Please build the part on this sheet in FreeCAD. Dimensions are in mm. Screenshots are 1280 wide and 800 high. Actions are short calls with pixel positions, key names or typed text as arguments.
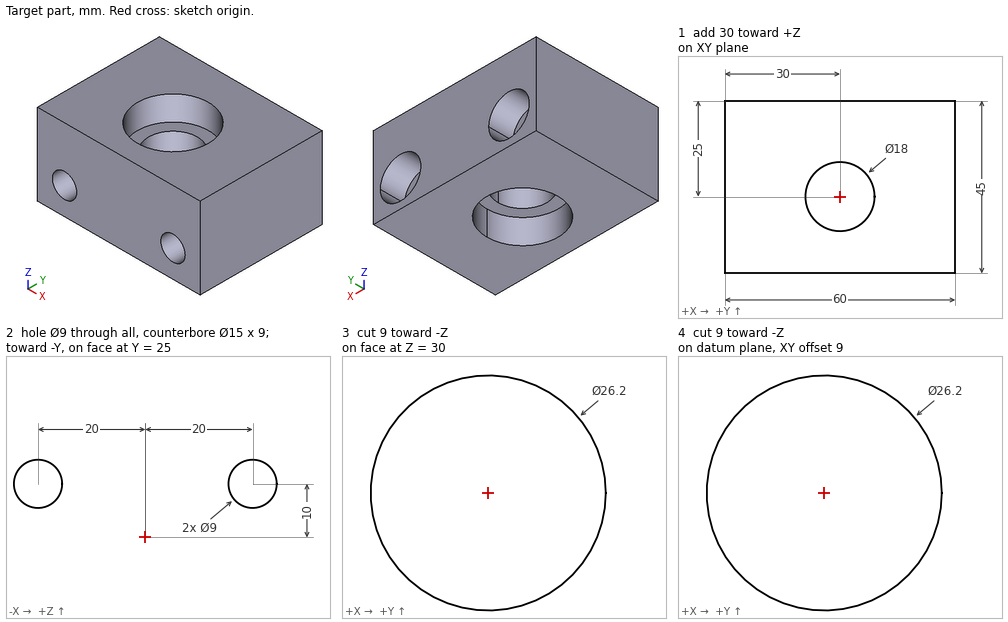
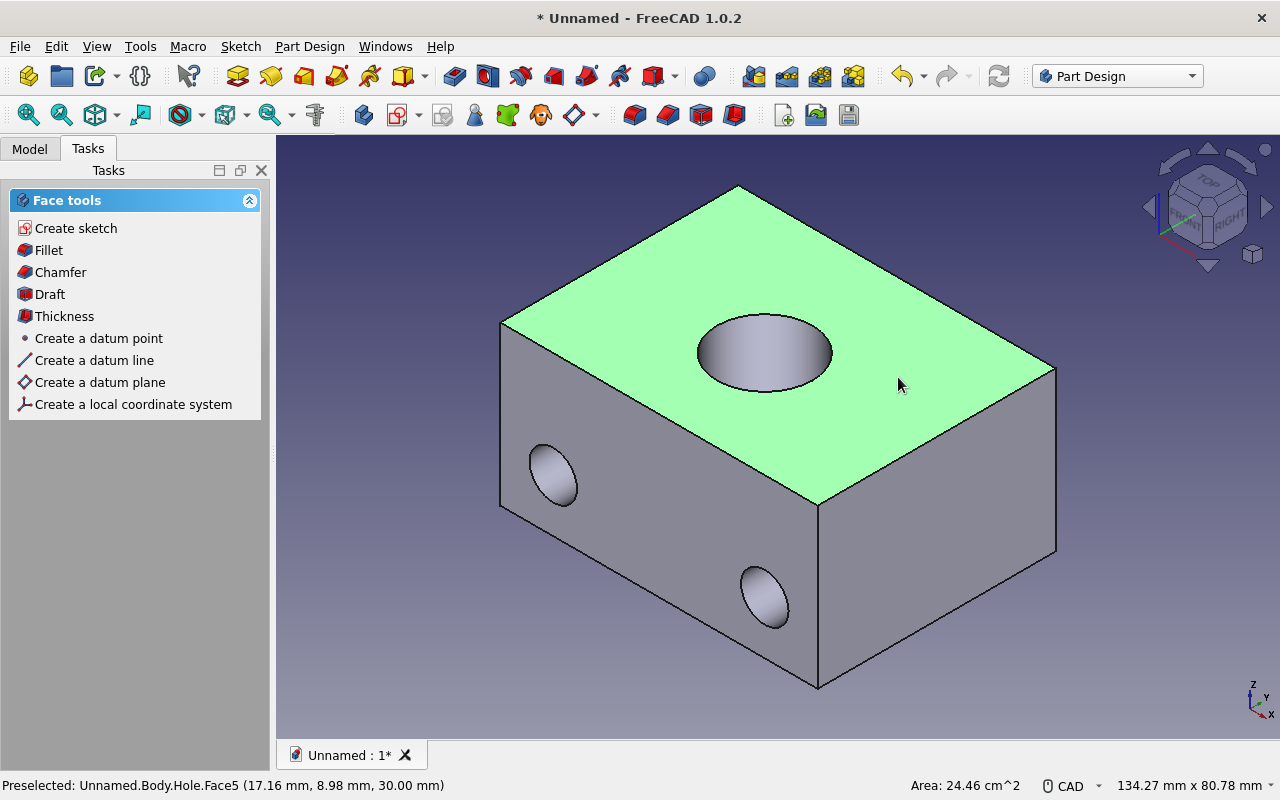
click(396, 116)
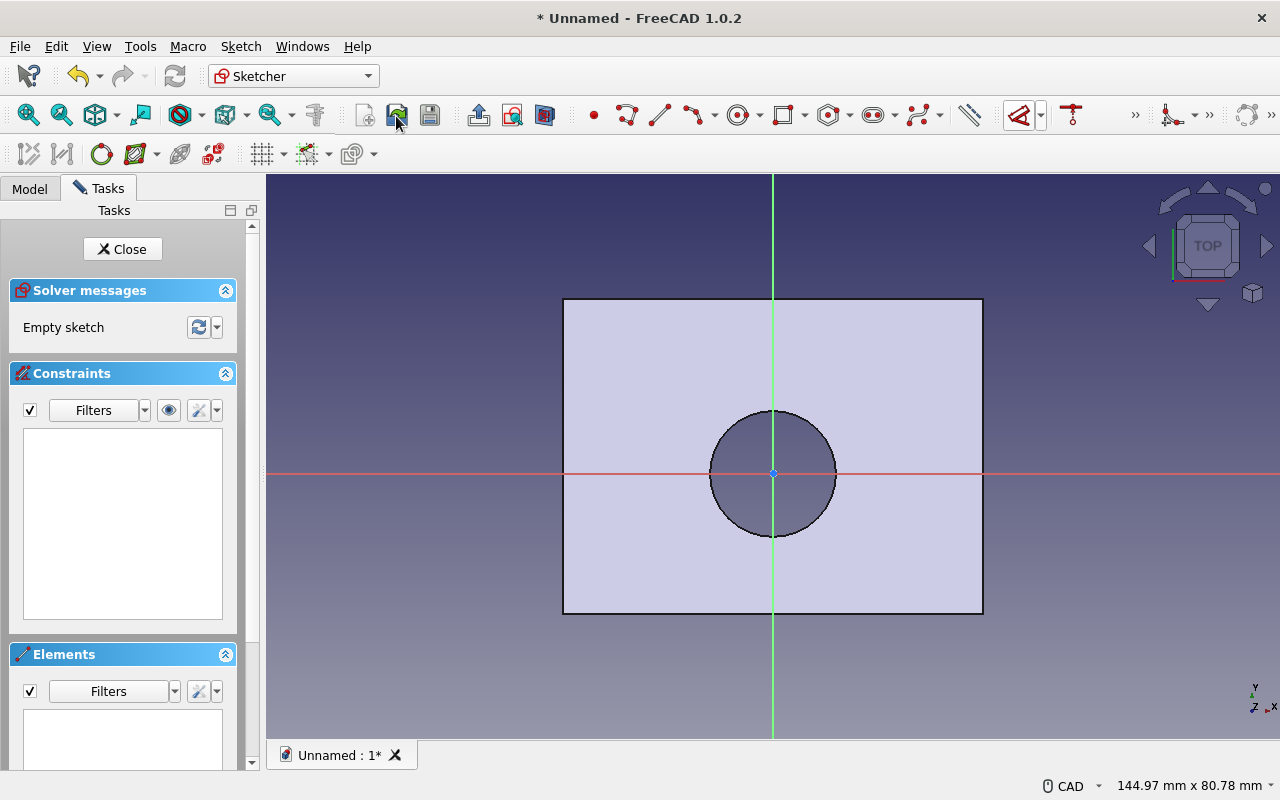
scroll(856, 495, up, 3)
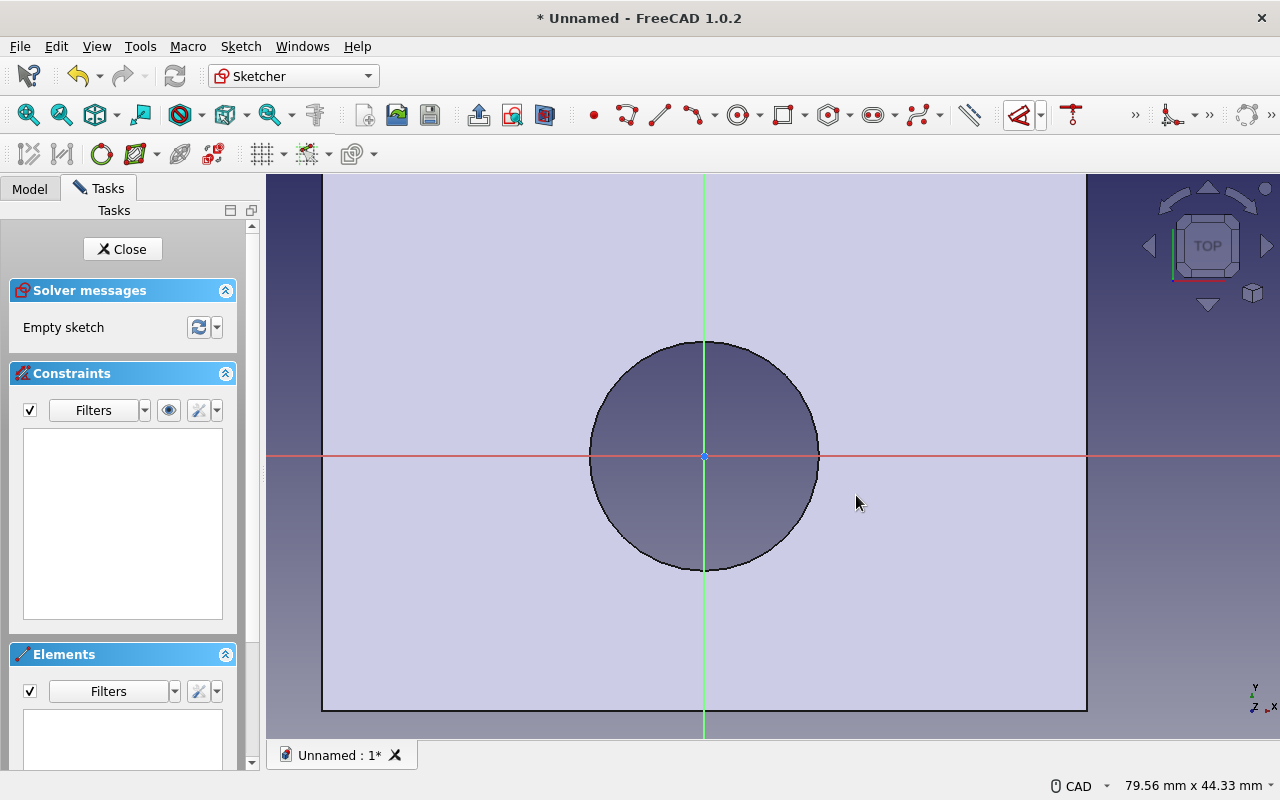
click(738, 116)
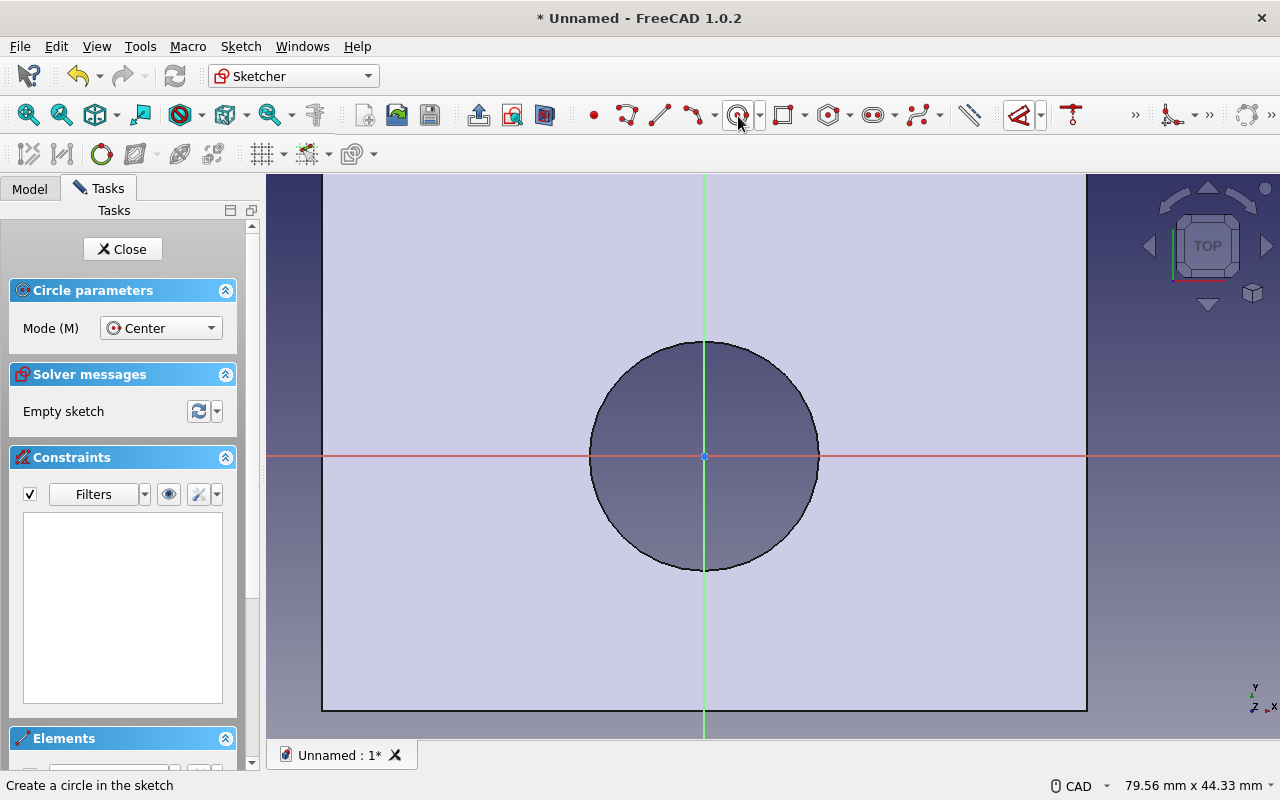
click(704, 456)
move(822, 338)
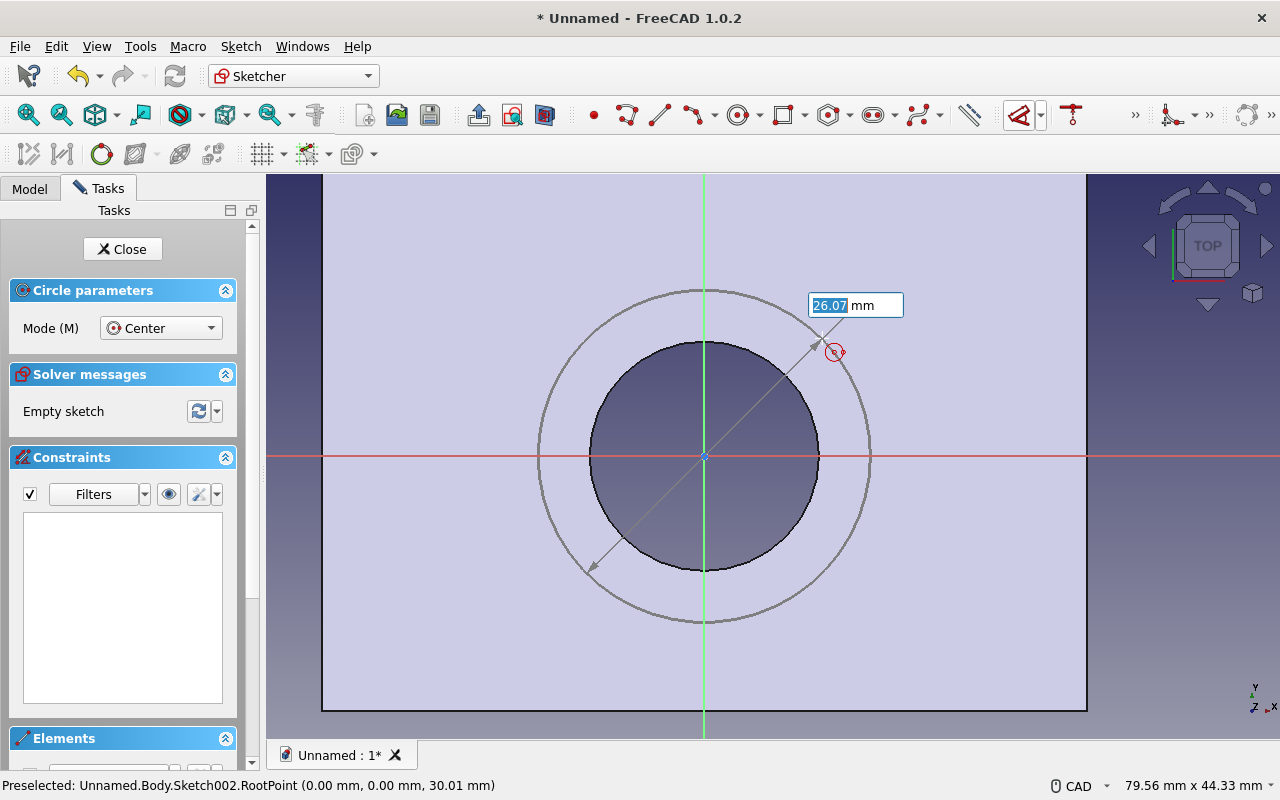
text(26.2)
key(Return)
key(Escape)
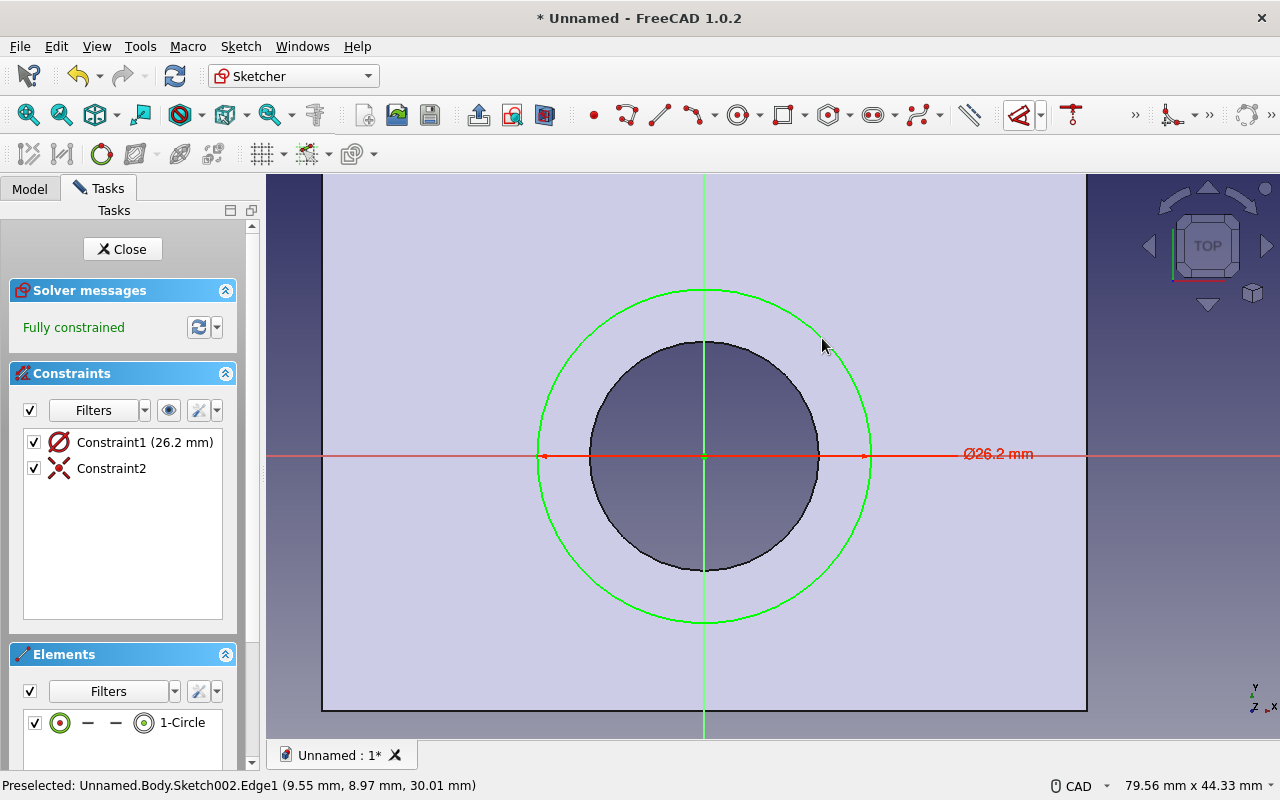
click(123, 249)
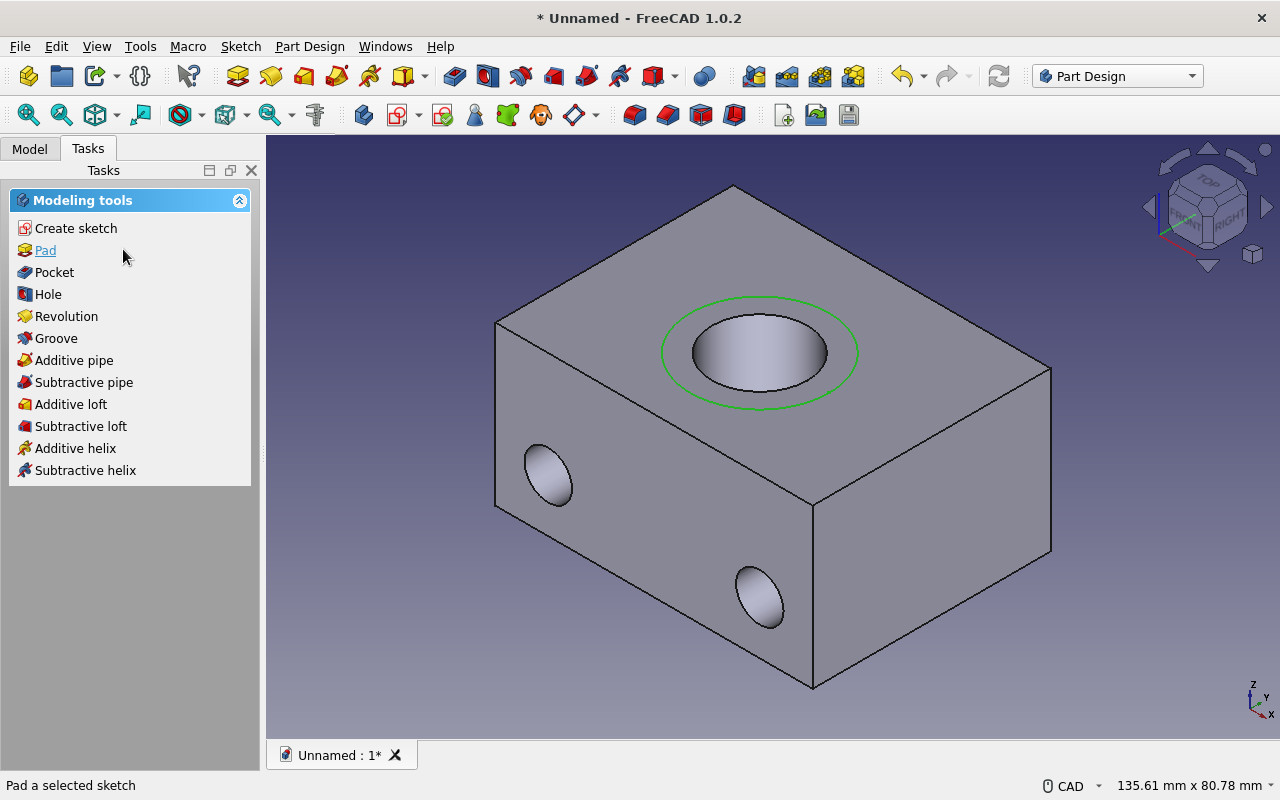
click(455, 76)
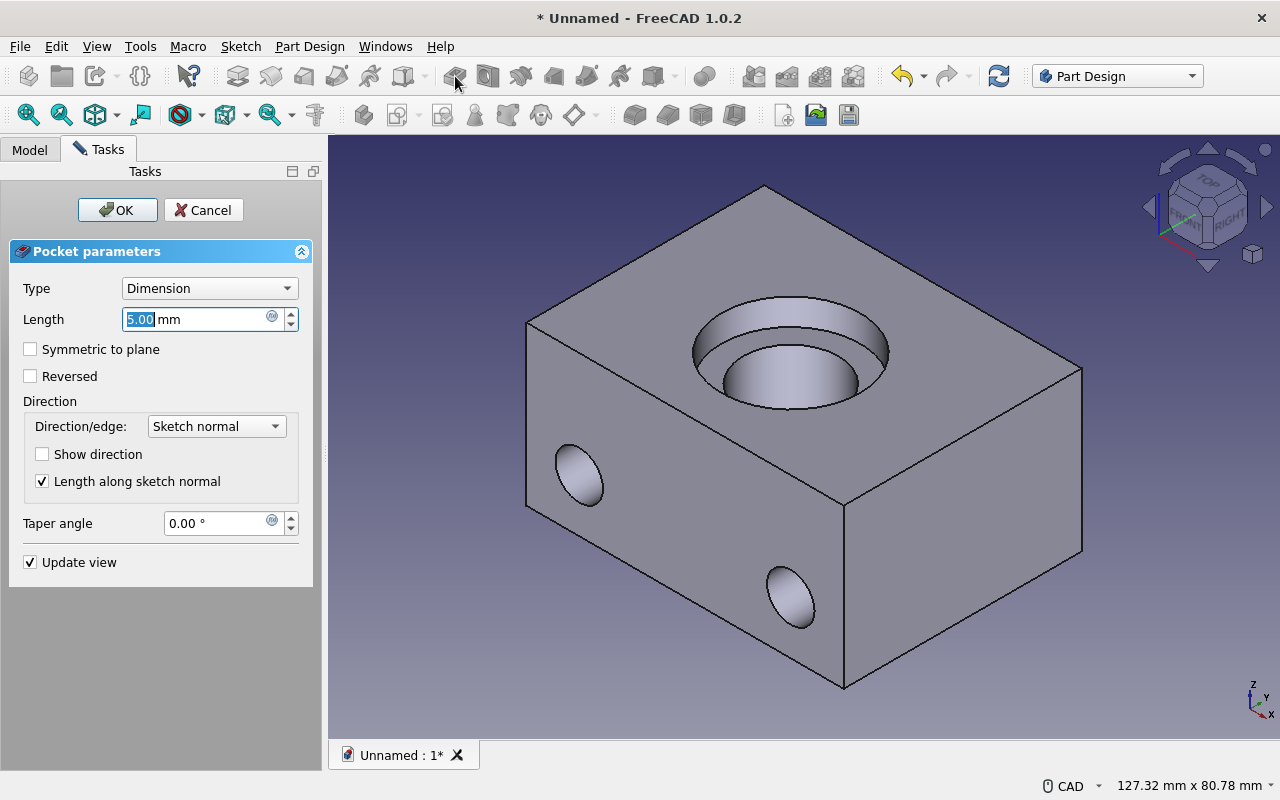
text(9)
key(Tab)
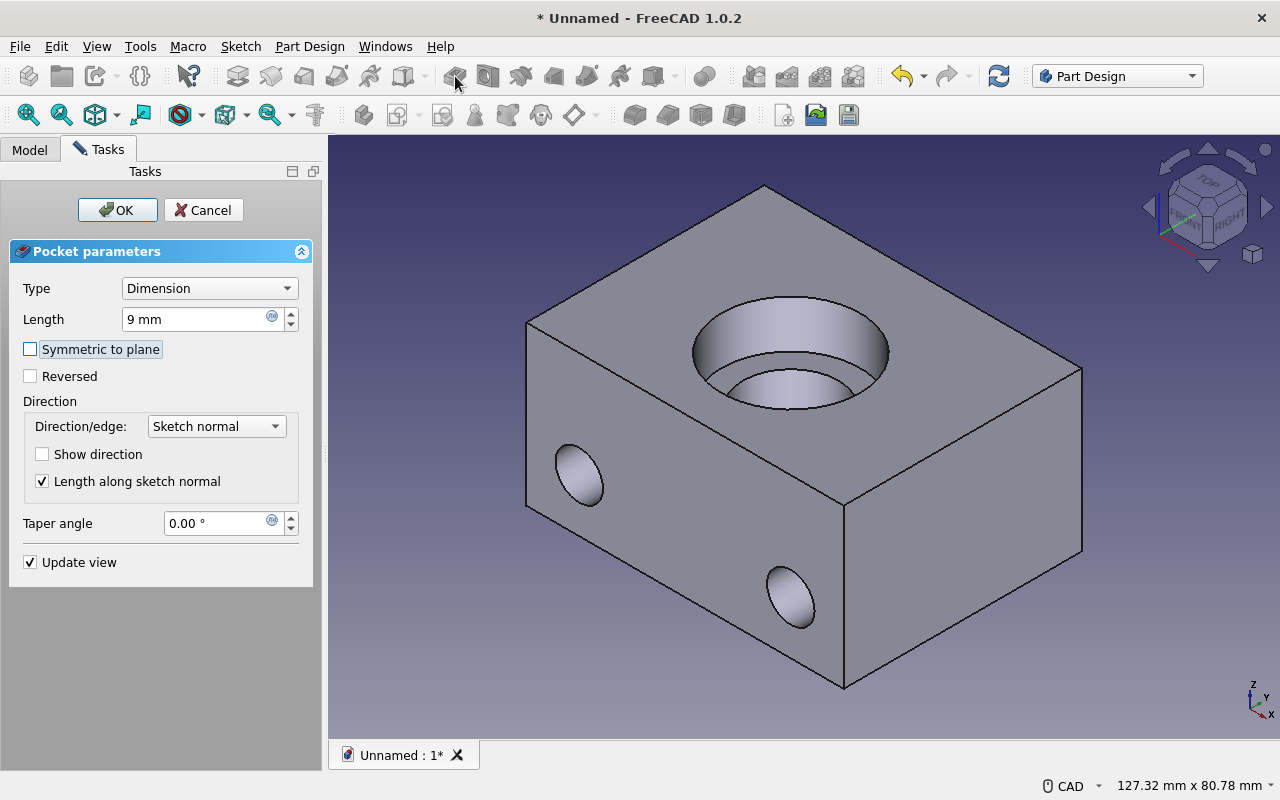
click(118, 210)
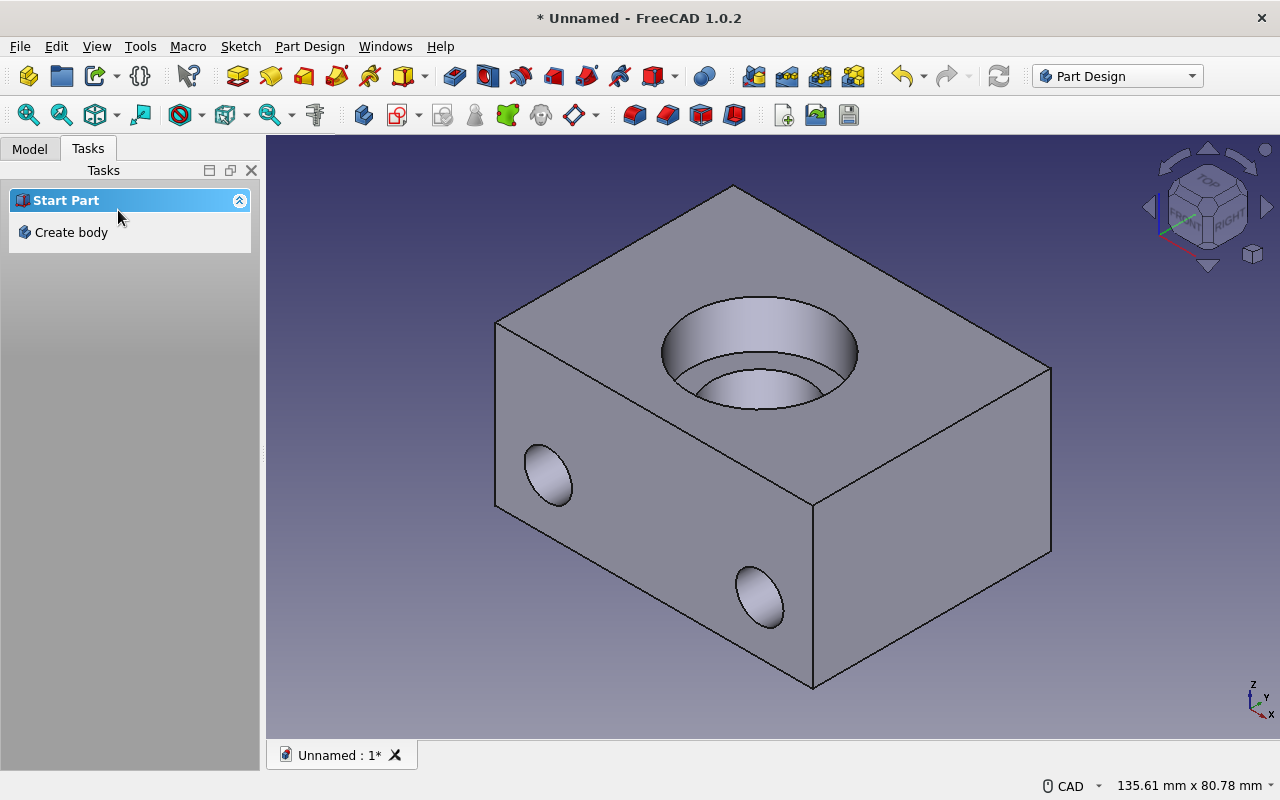
click(30, 148)